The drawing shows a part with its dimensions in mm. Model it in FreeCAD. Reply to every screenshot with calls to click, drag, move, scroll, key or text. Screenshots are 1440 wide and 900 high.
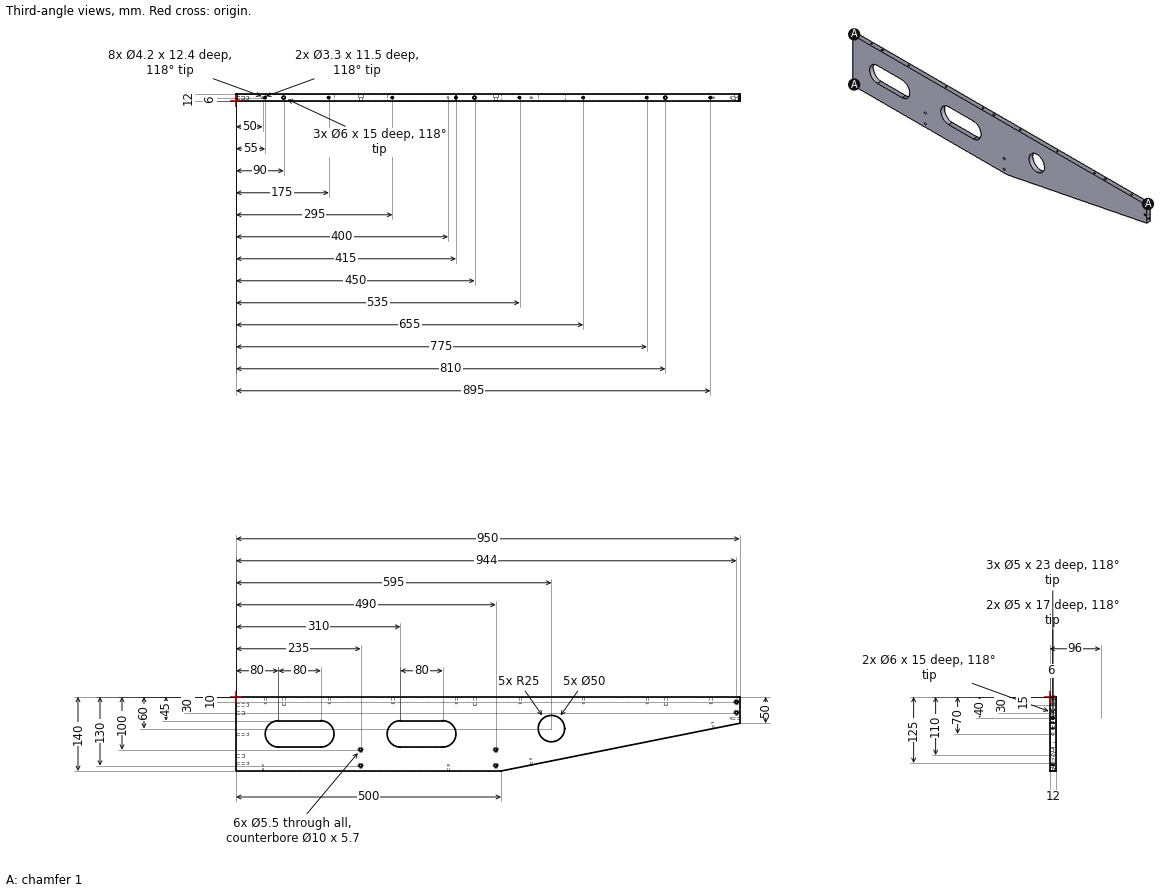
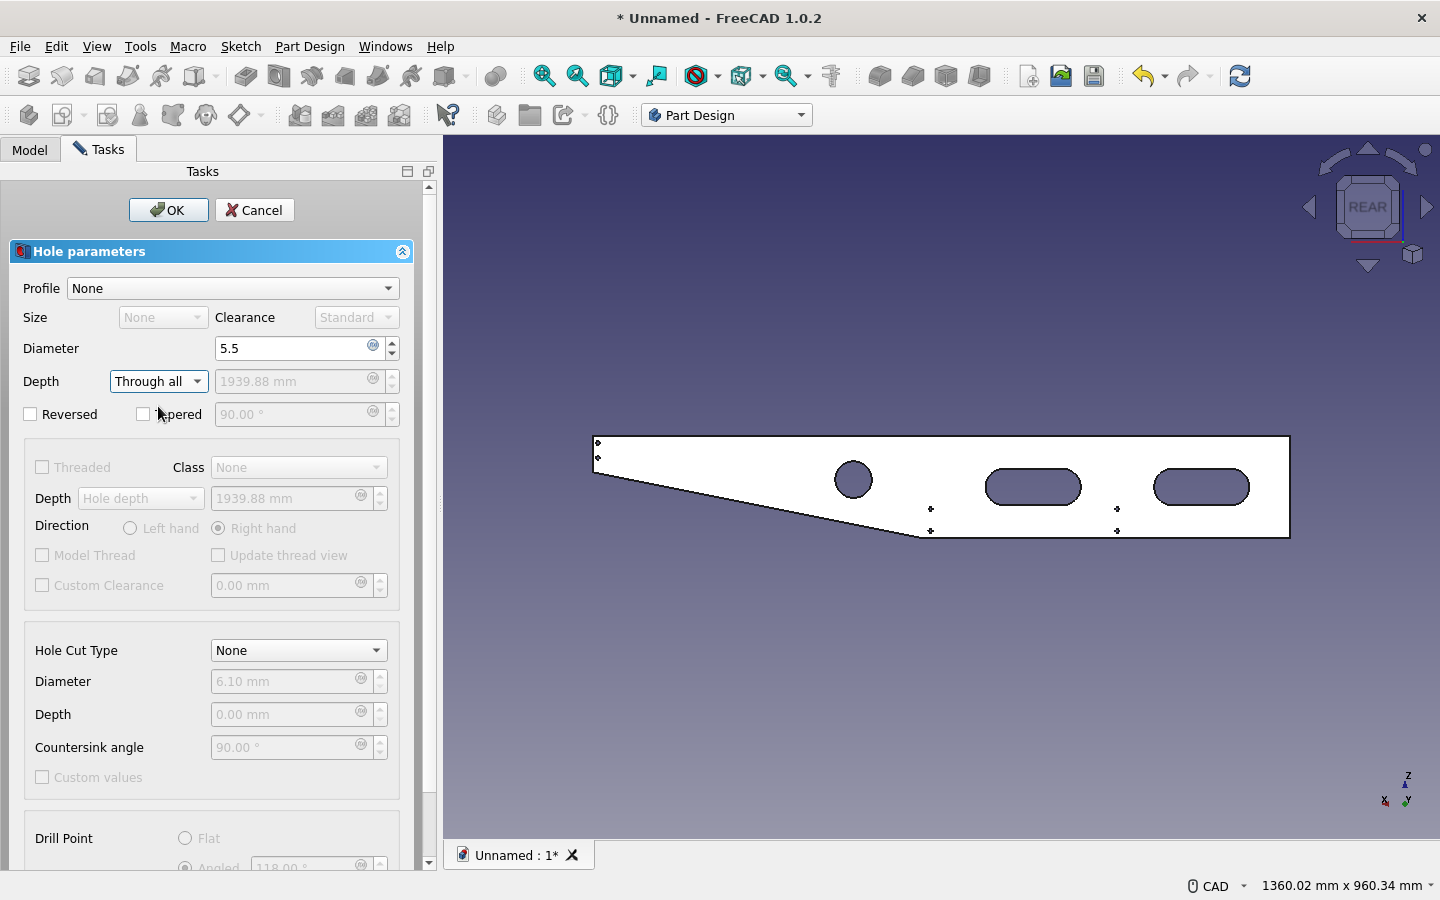
click(300, 650)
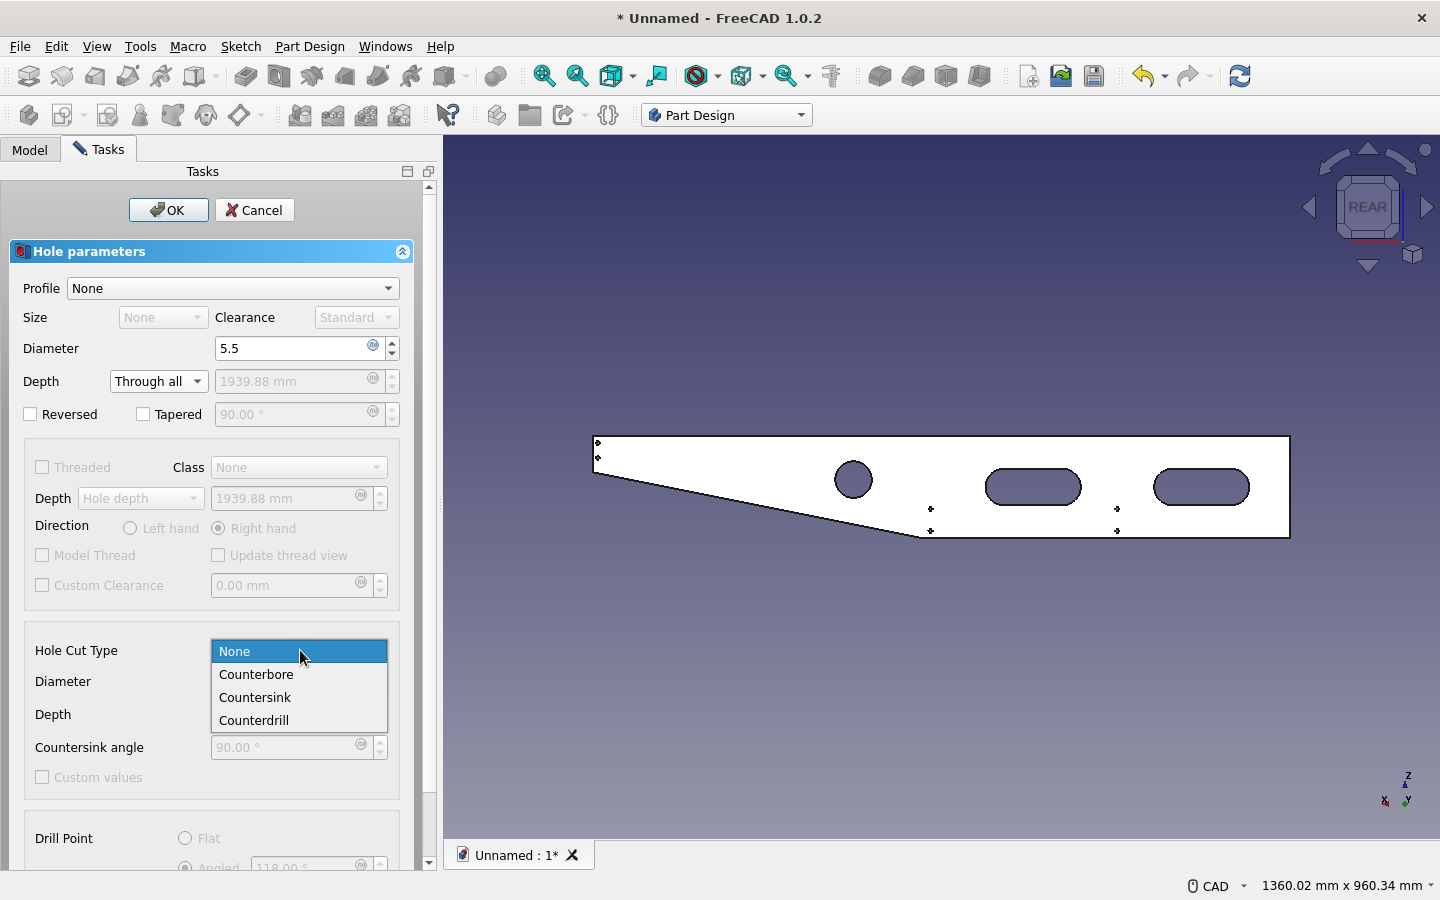
click(298, 674)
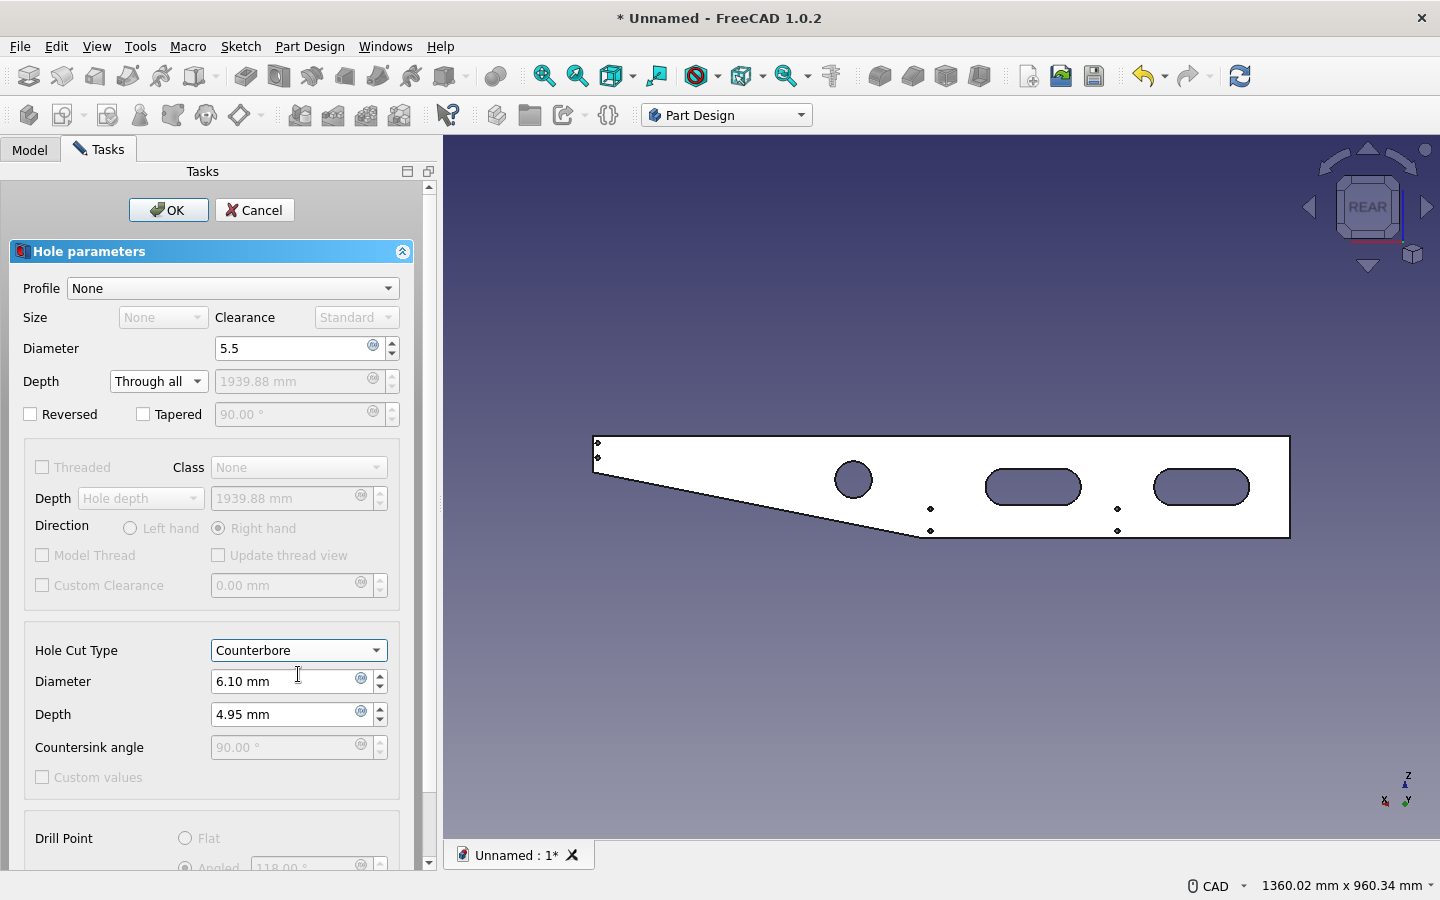
triple_click(292, 682)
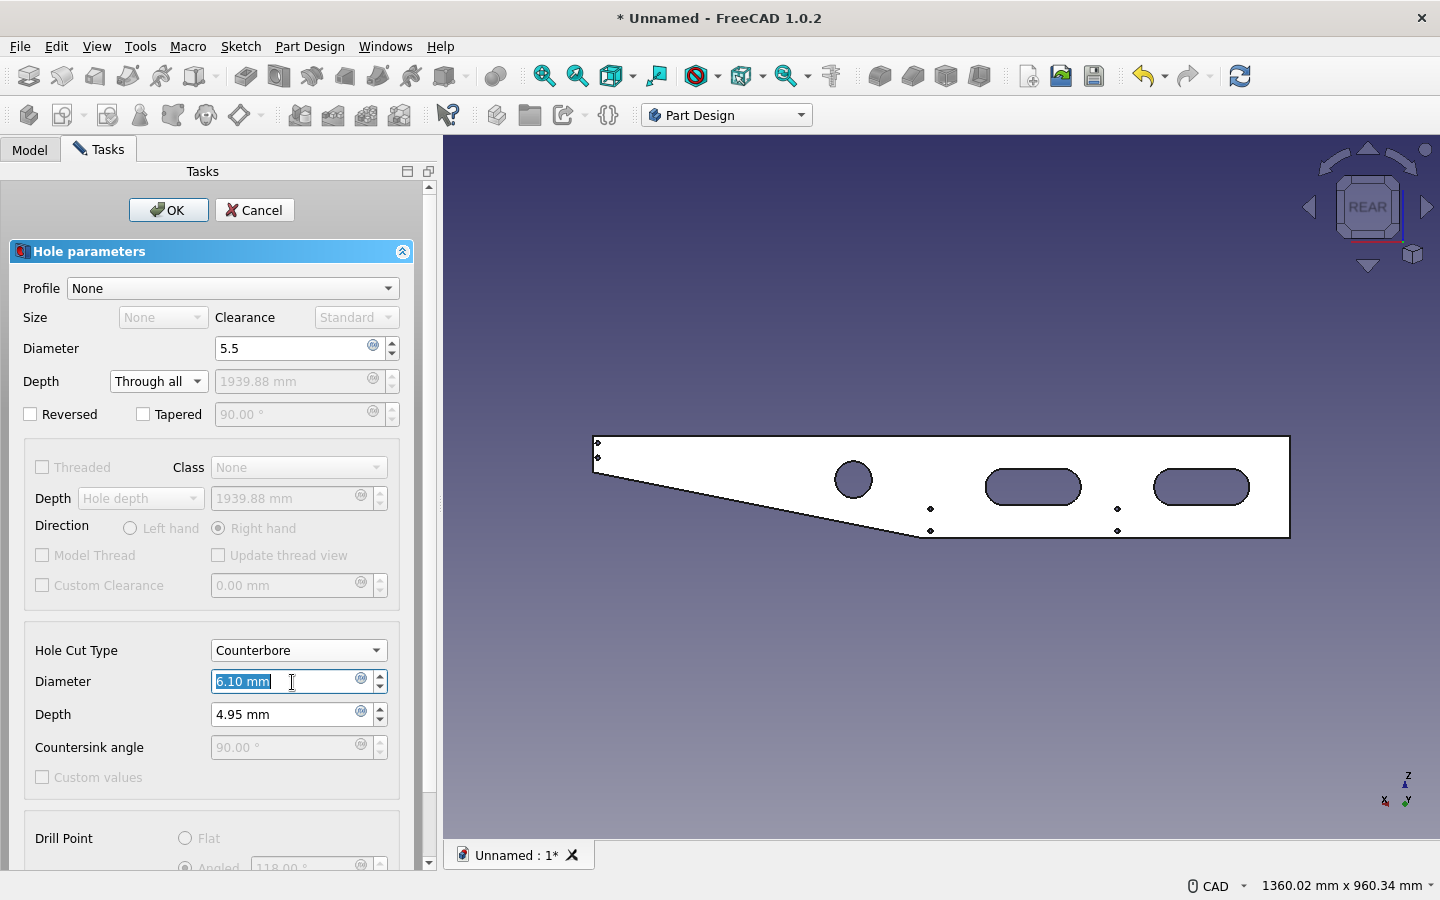
text(10)
key(Tab)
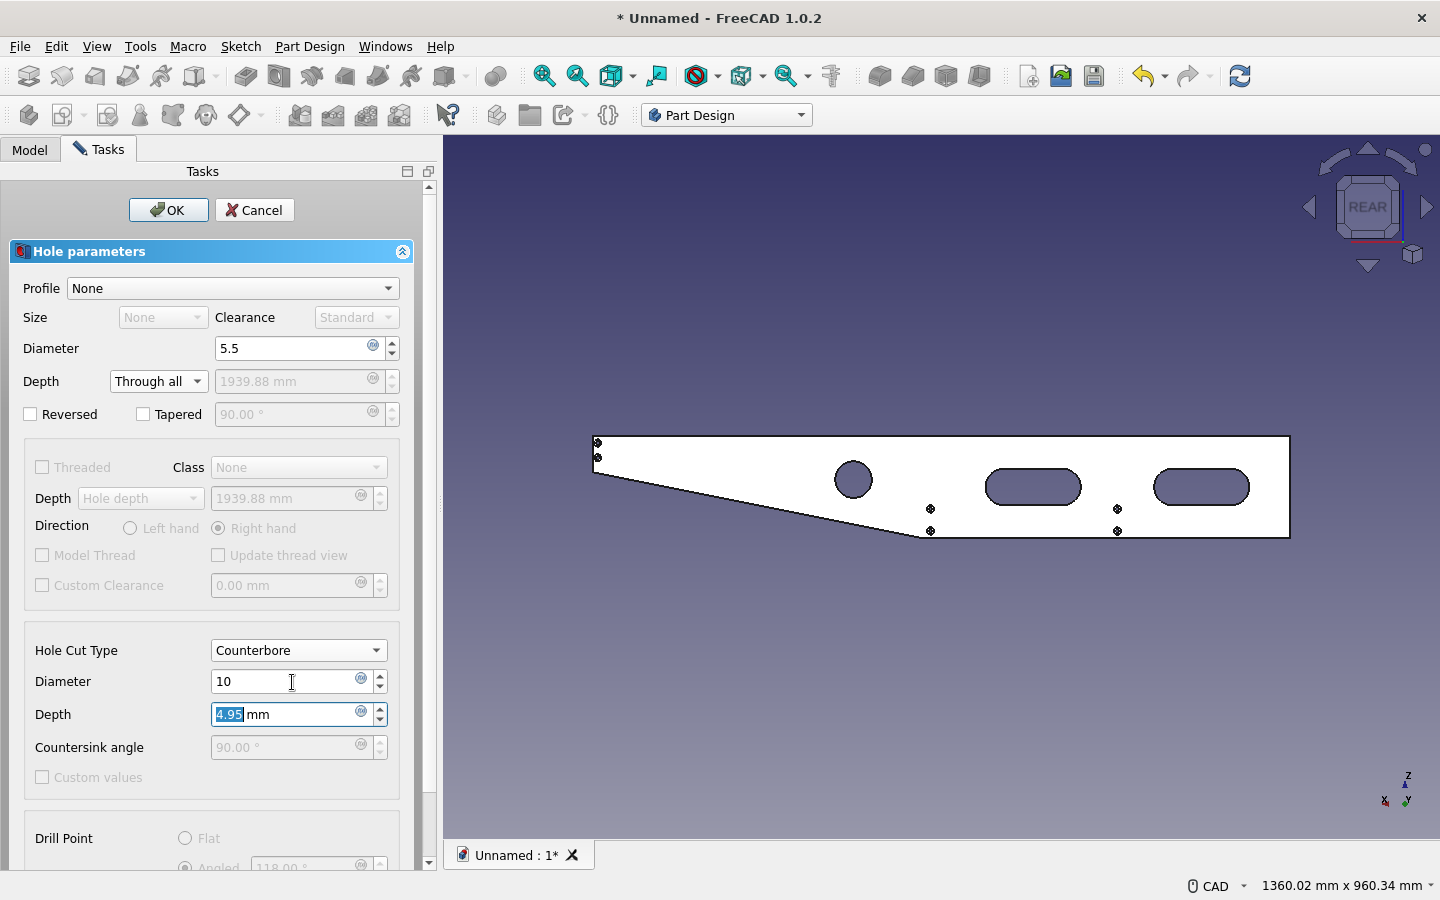
text(5.7)
key(Tab)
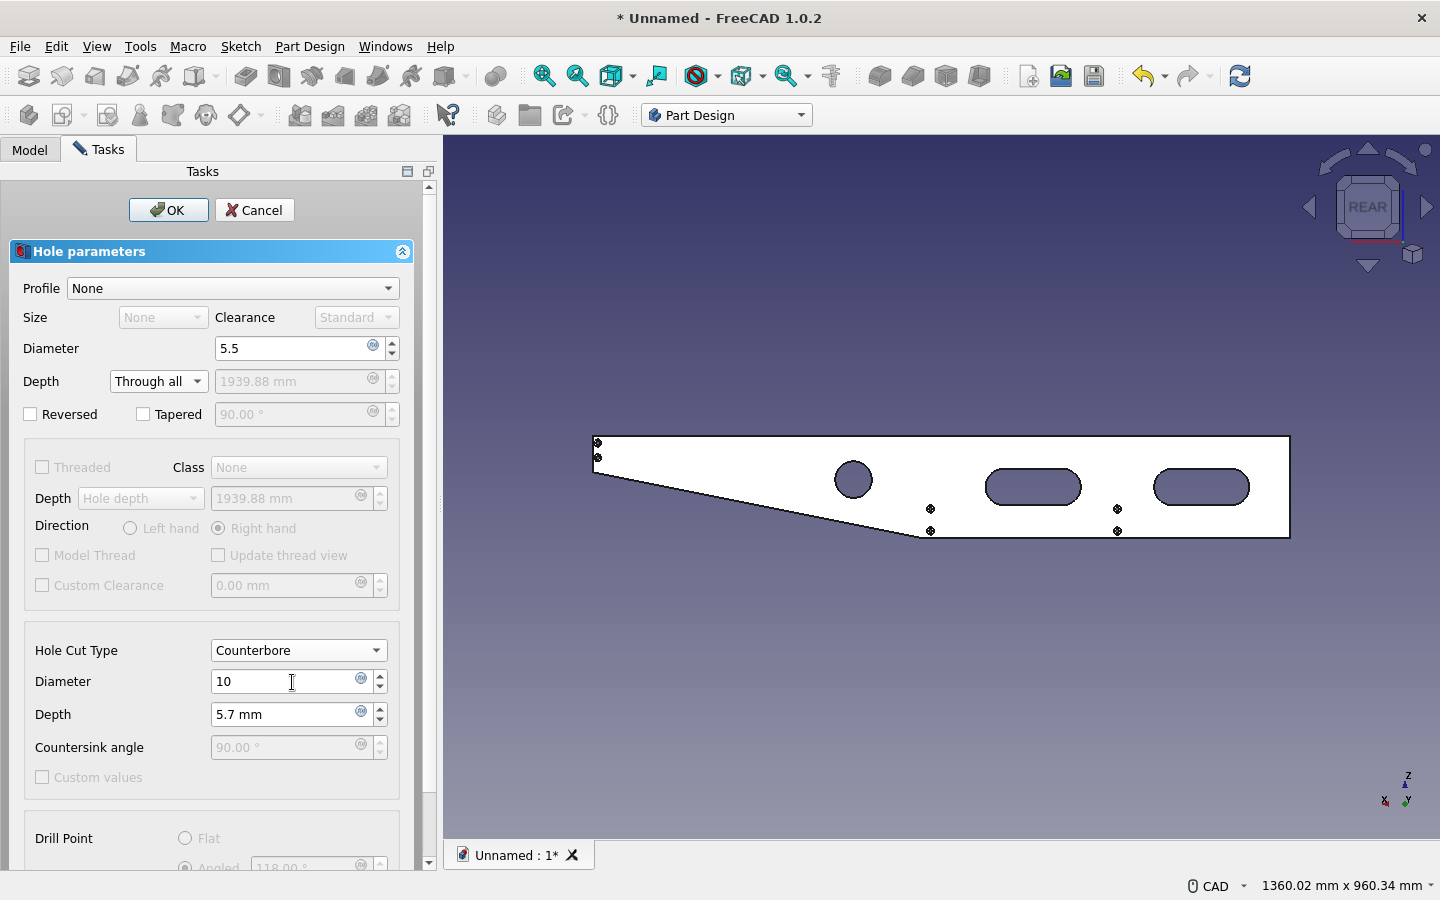
click(169, 210)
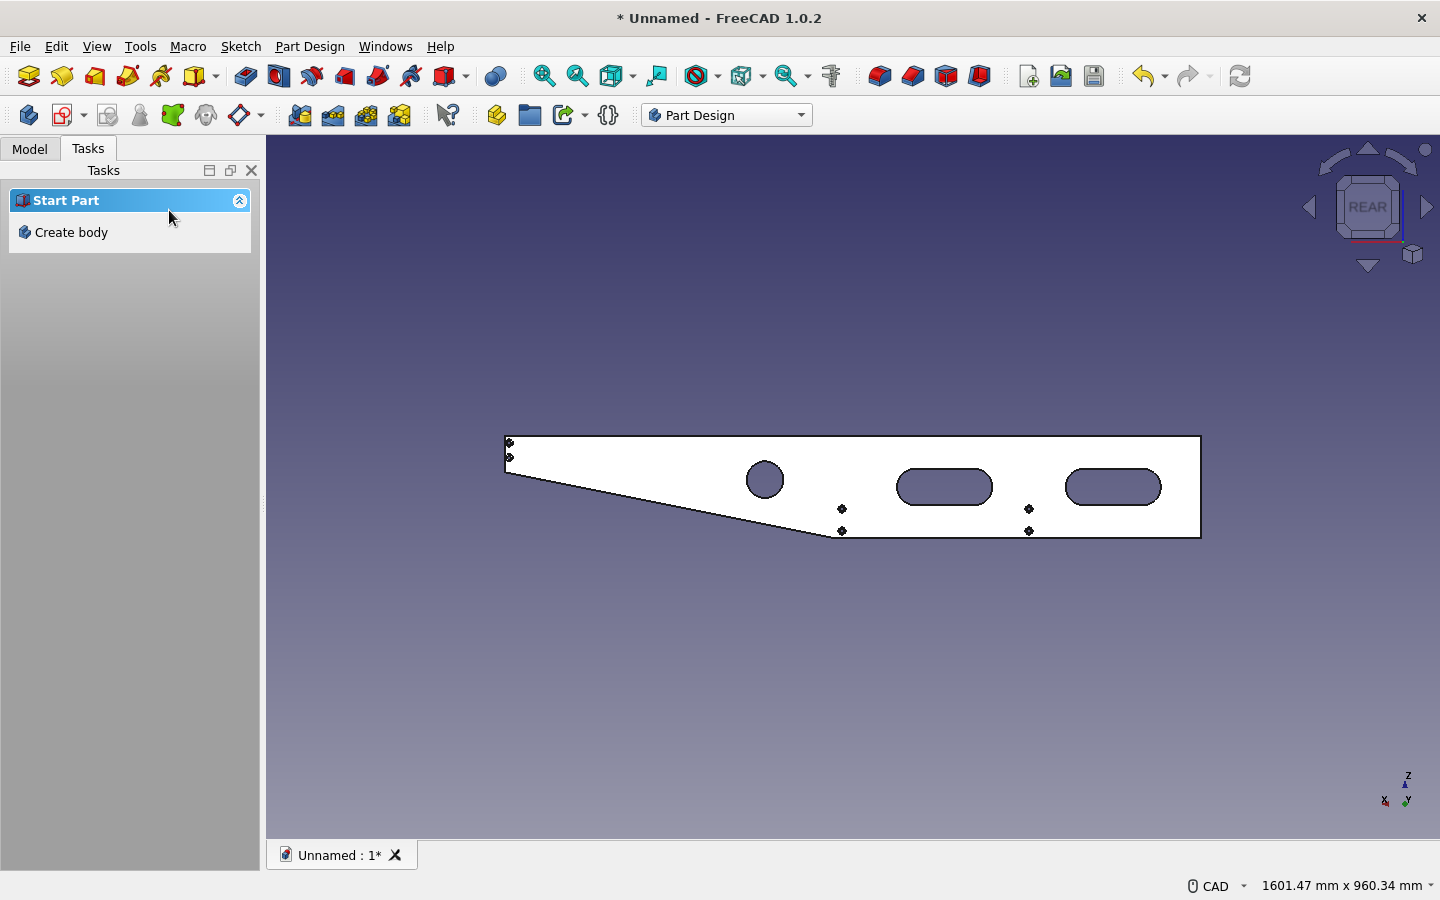
scroll(505, 435, up, 8)